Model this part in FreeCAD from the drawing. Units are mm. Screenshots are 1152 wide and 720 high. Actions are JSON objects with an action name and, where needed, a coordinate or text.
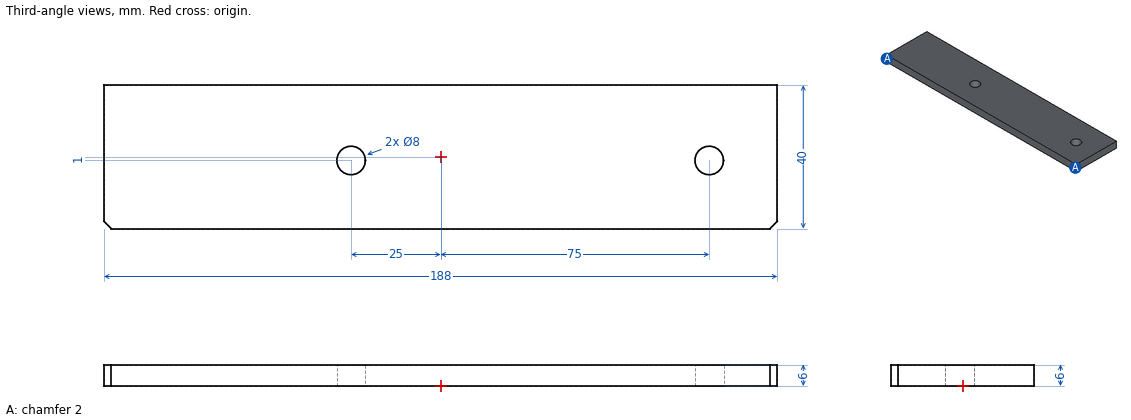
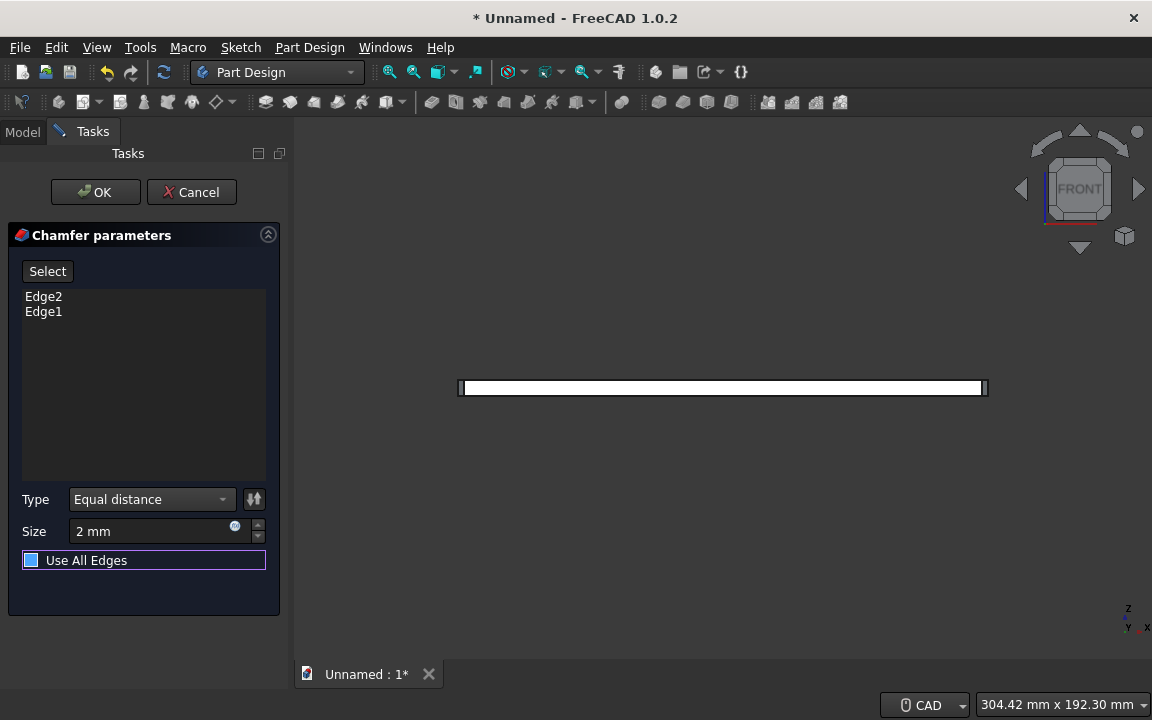
{"action": "left_click", "coordinate": [96, 192]}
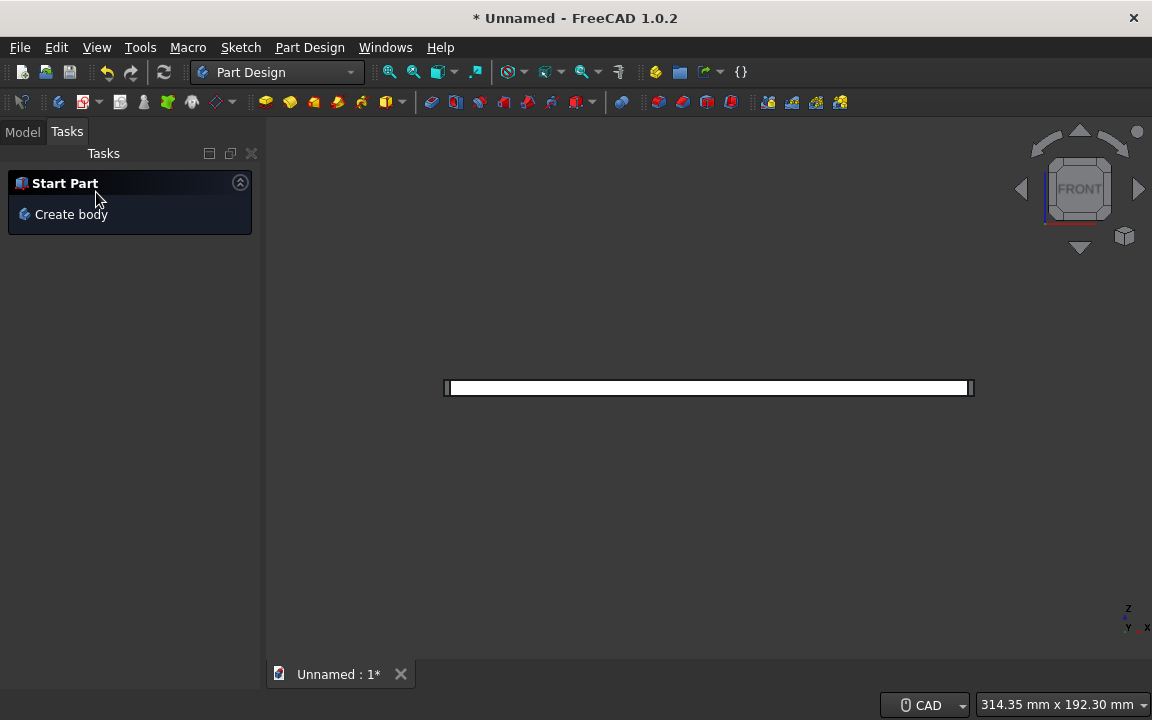
{"action": "key", "text": "0"}